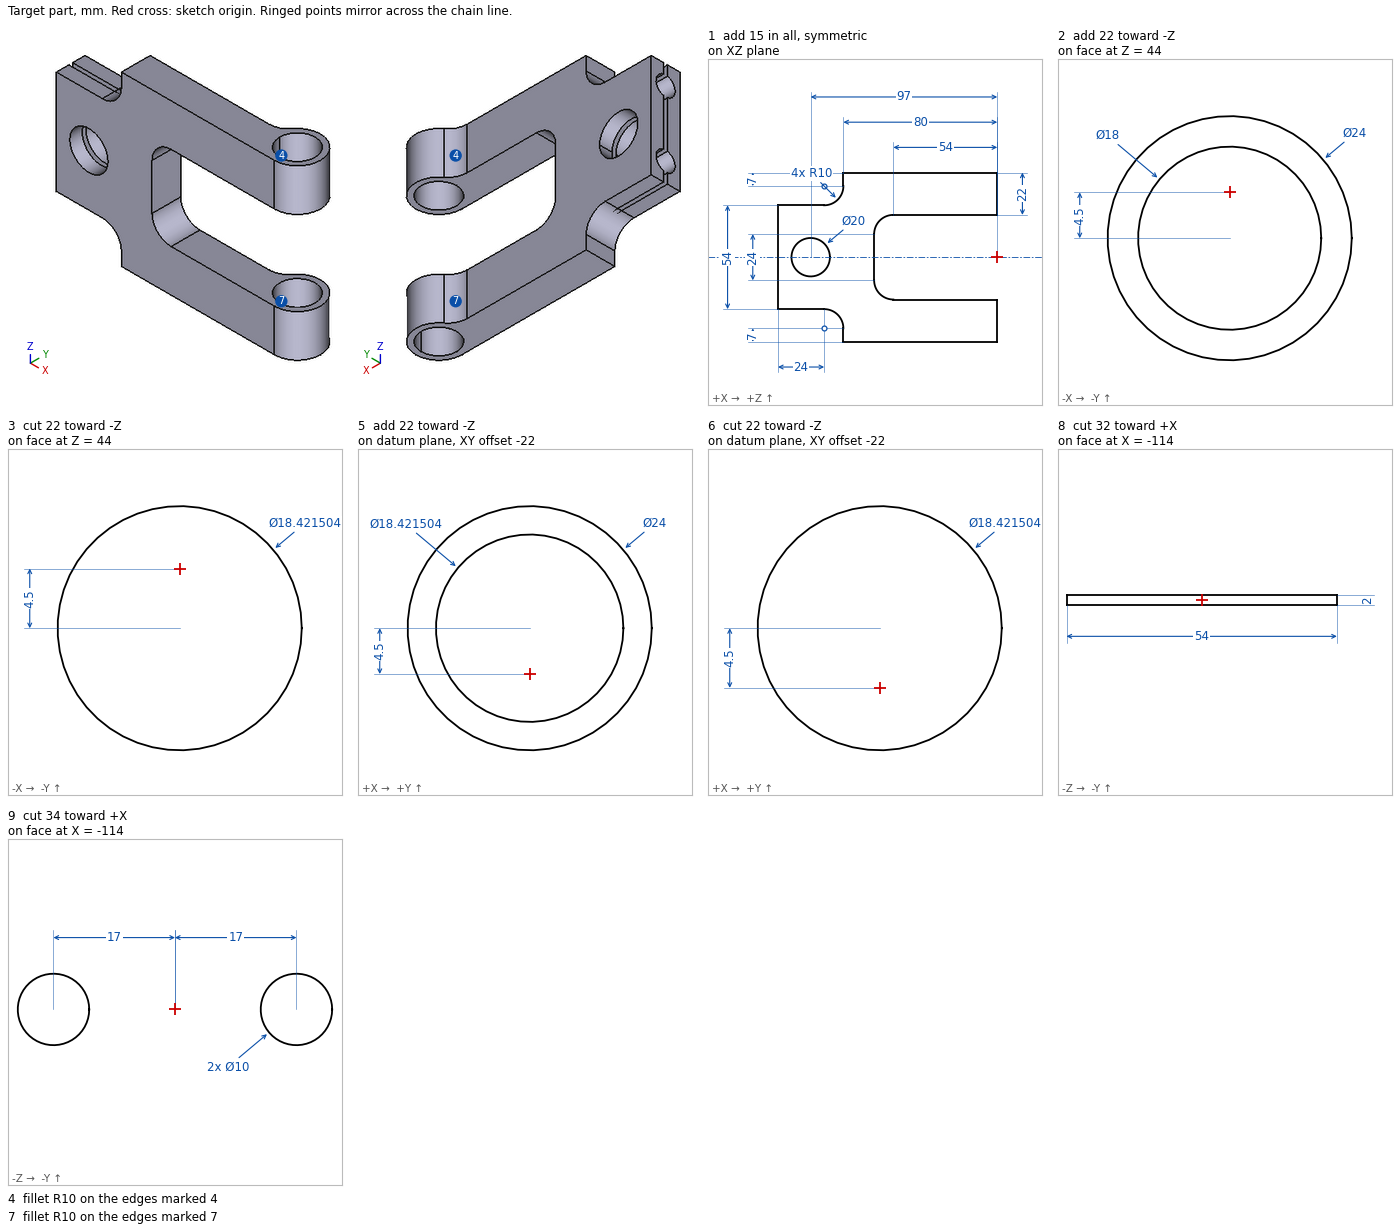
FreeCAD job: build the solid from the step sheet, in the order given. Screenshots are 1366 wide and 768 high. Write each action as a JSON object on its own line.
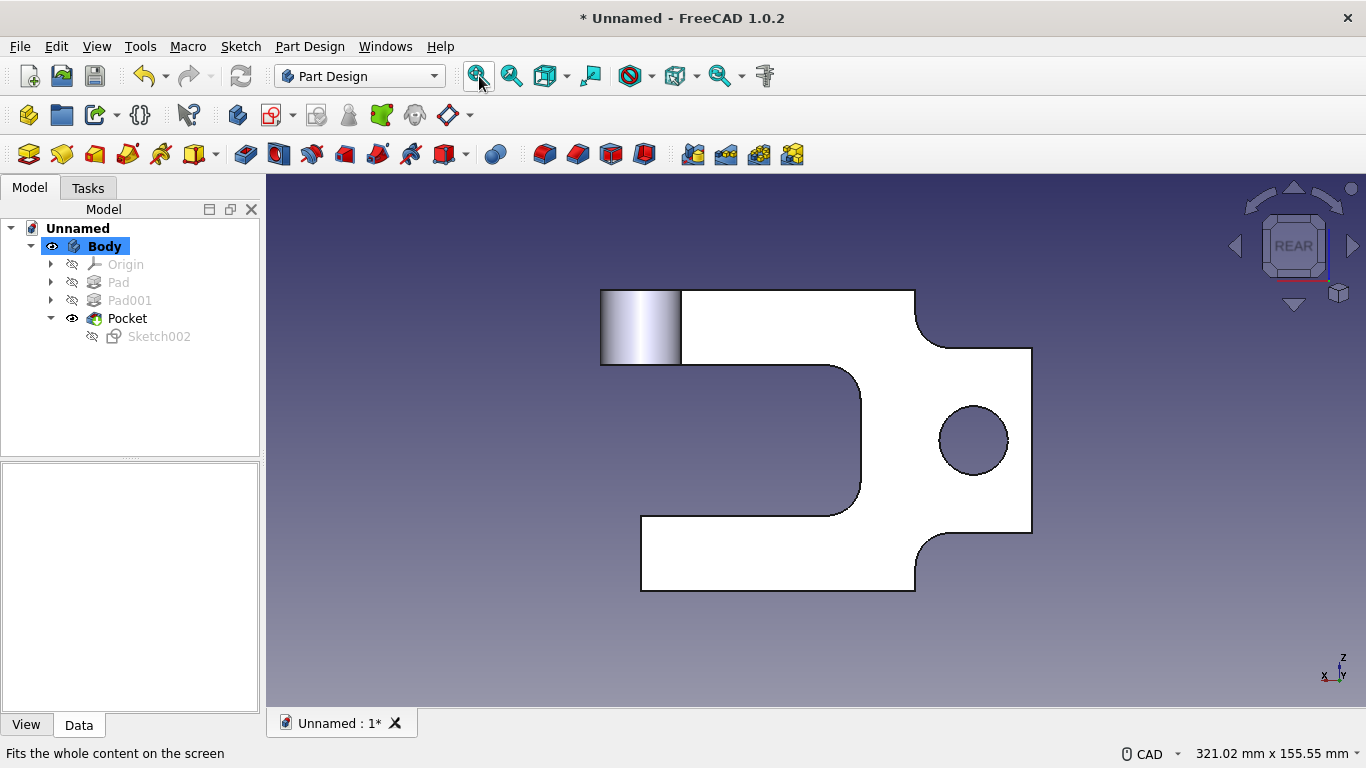
{"action": "key", "text": "6"}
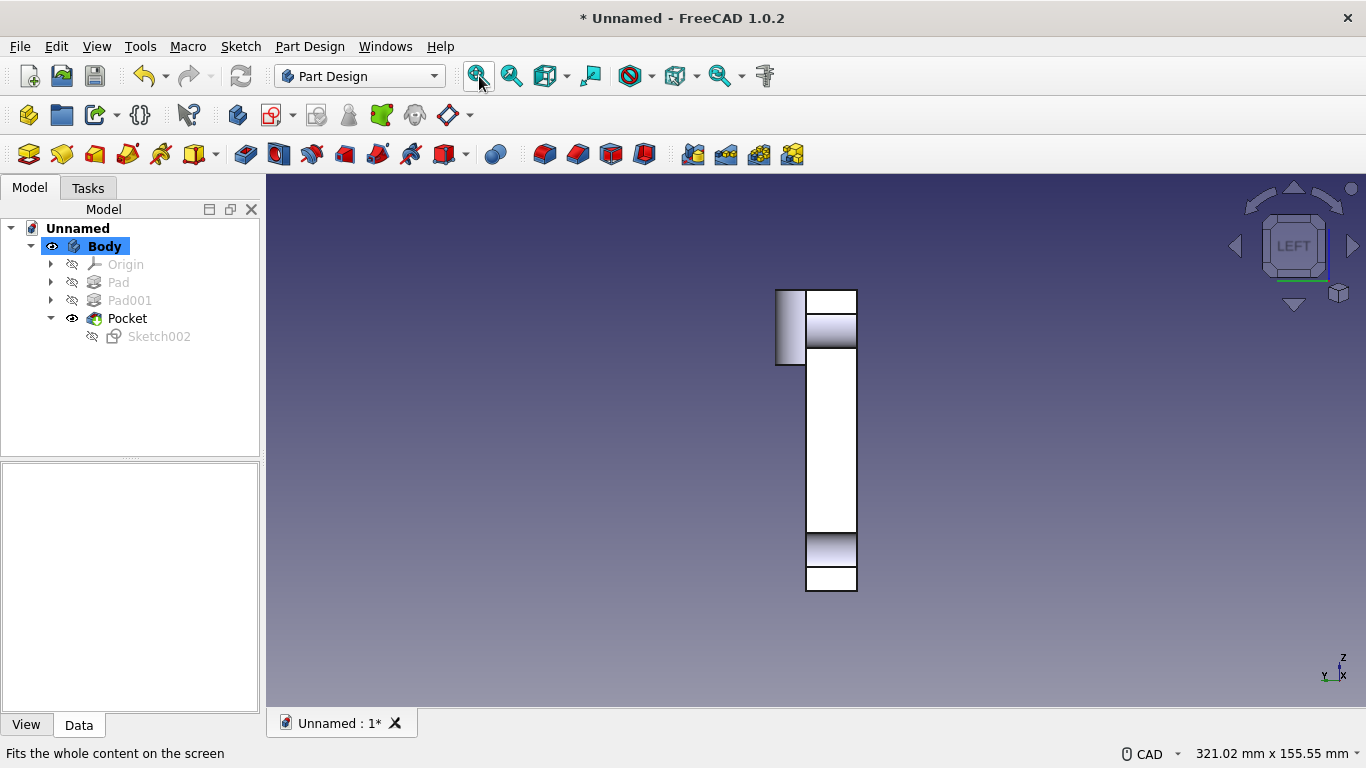
{"action": "key", "text": "v 3"}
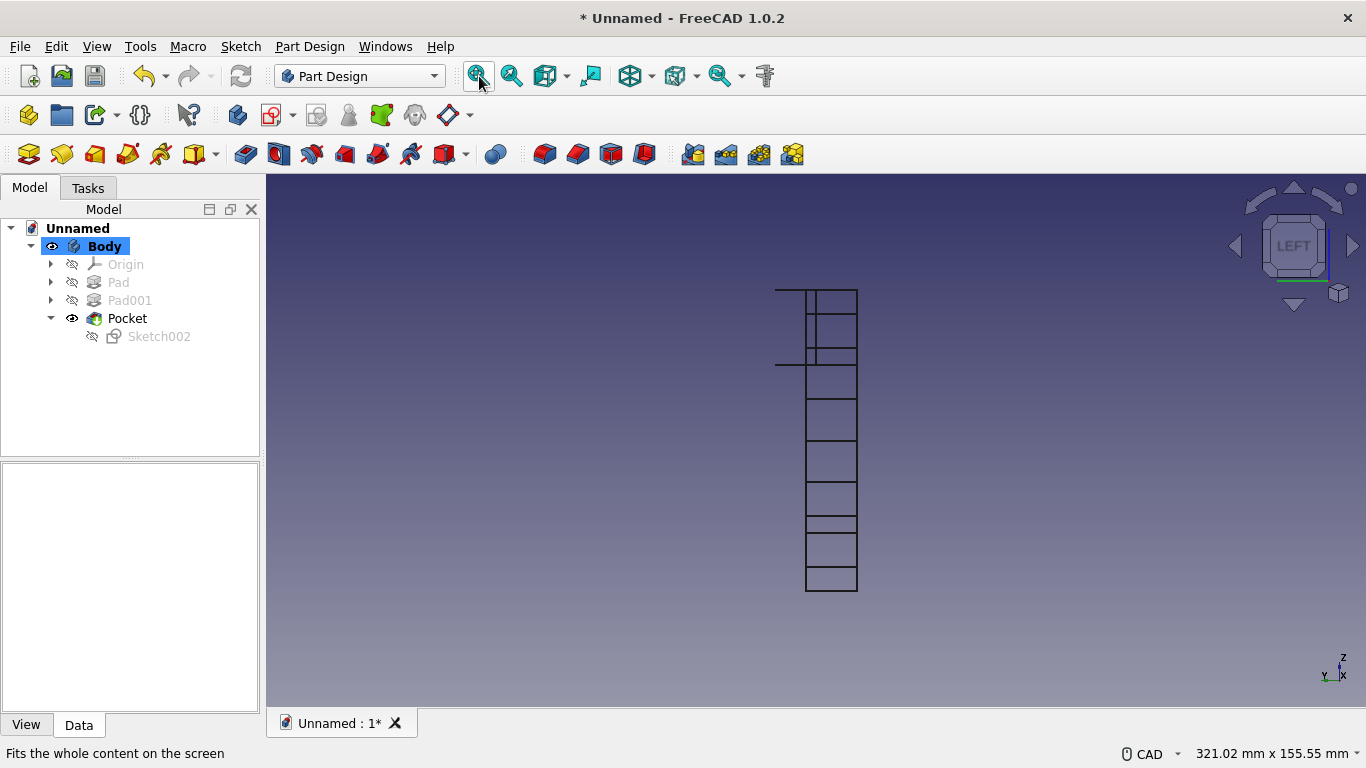
{"action": "key", "text": "0"}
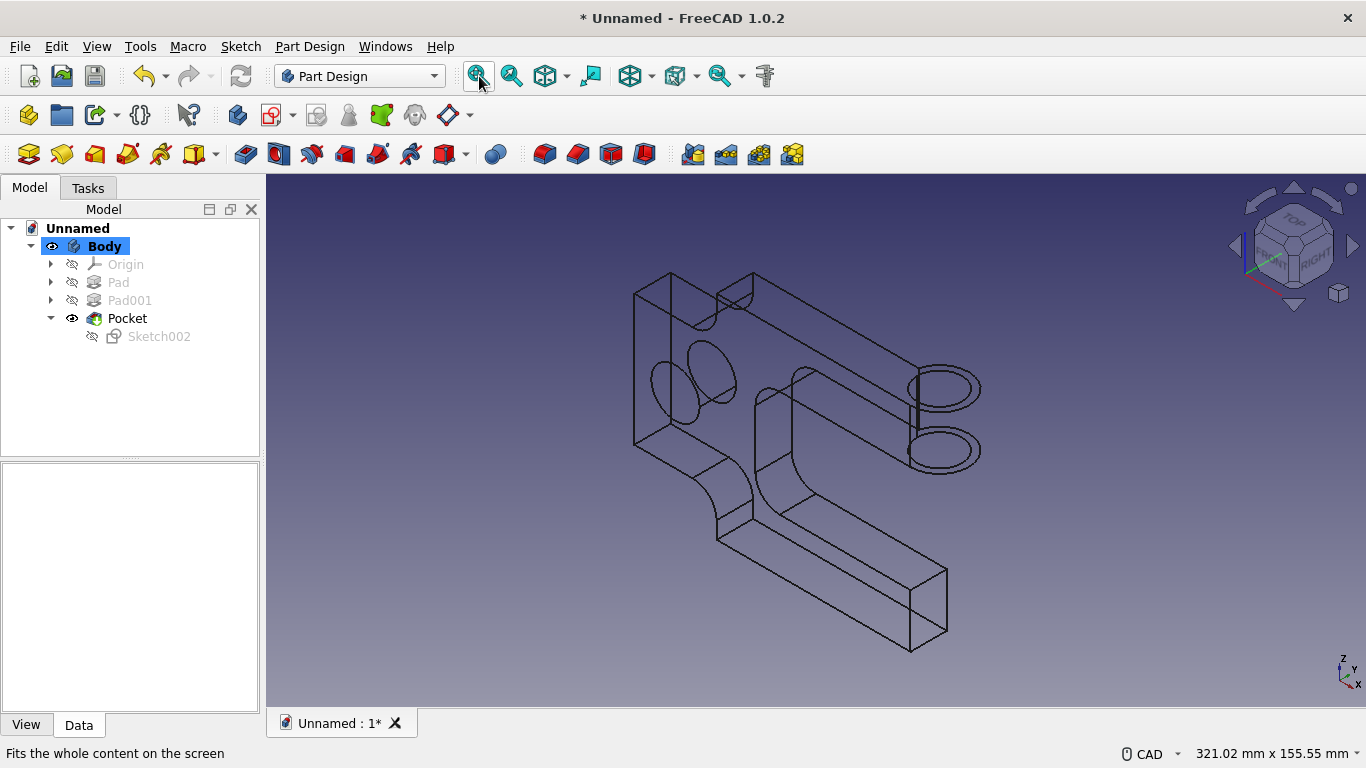
{"action": "key", "text": "2"}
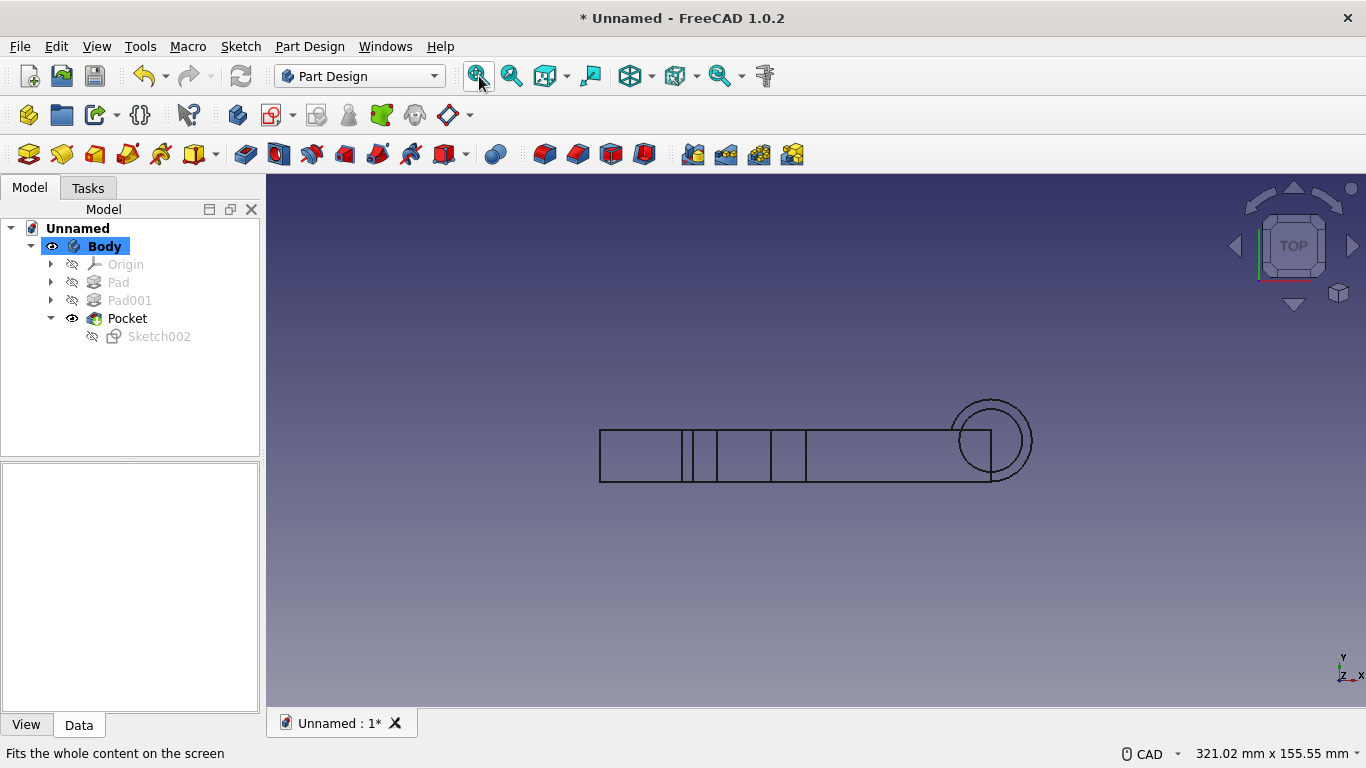
{"action": "left_click", "coordinate": [479, 76]}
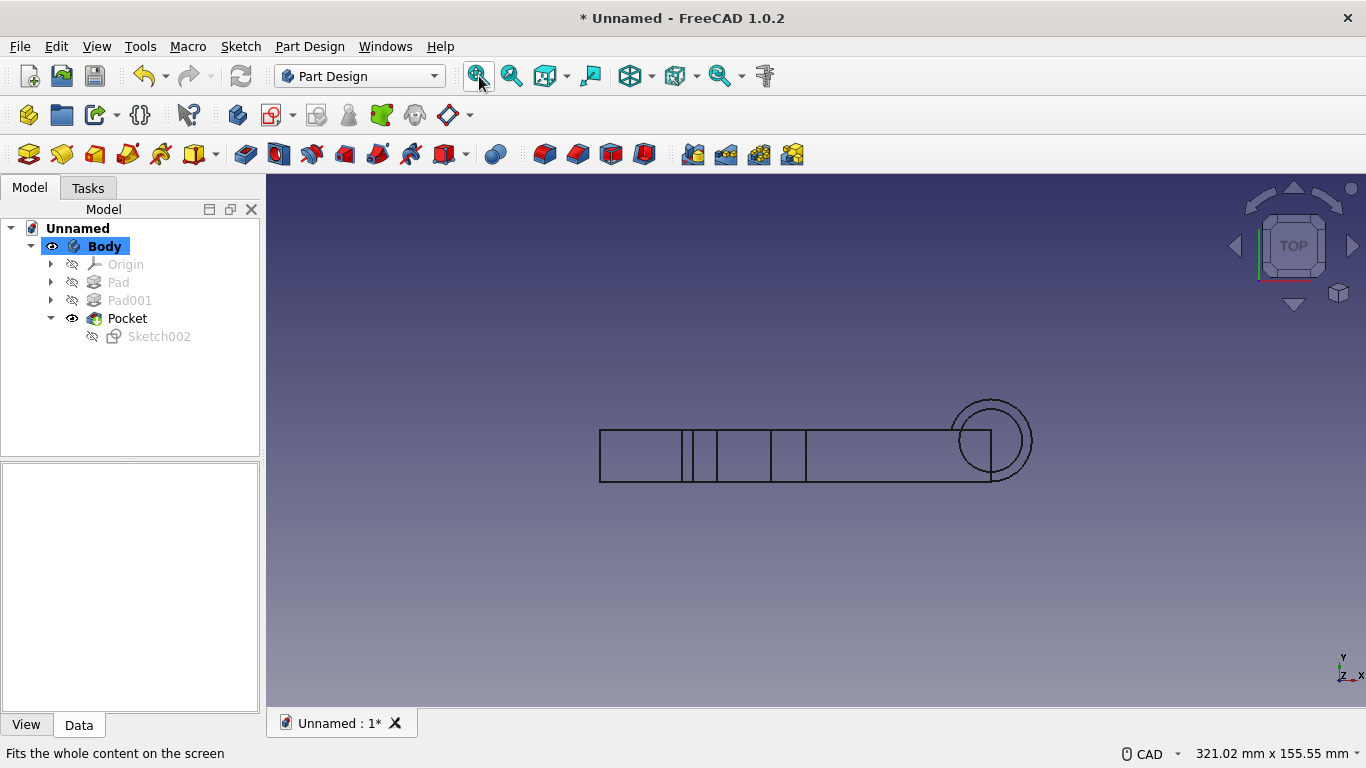
{"action": "key", "text": "1"}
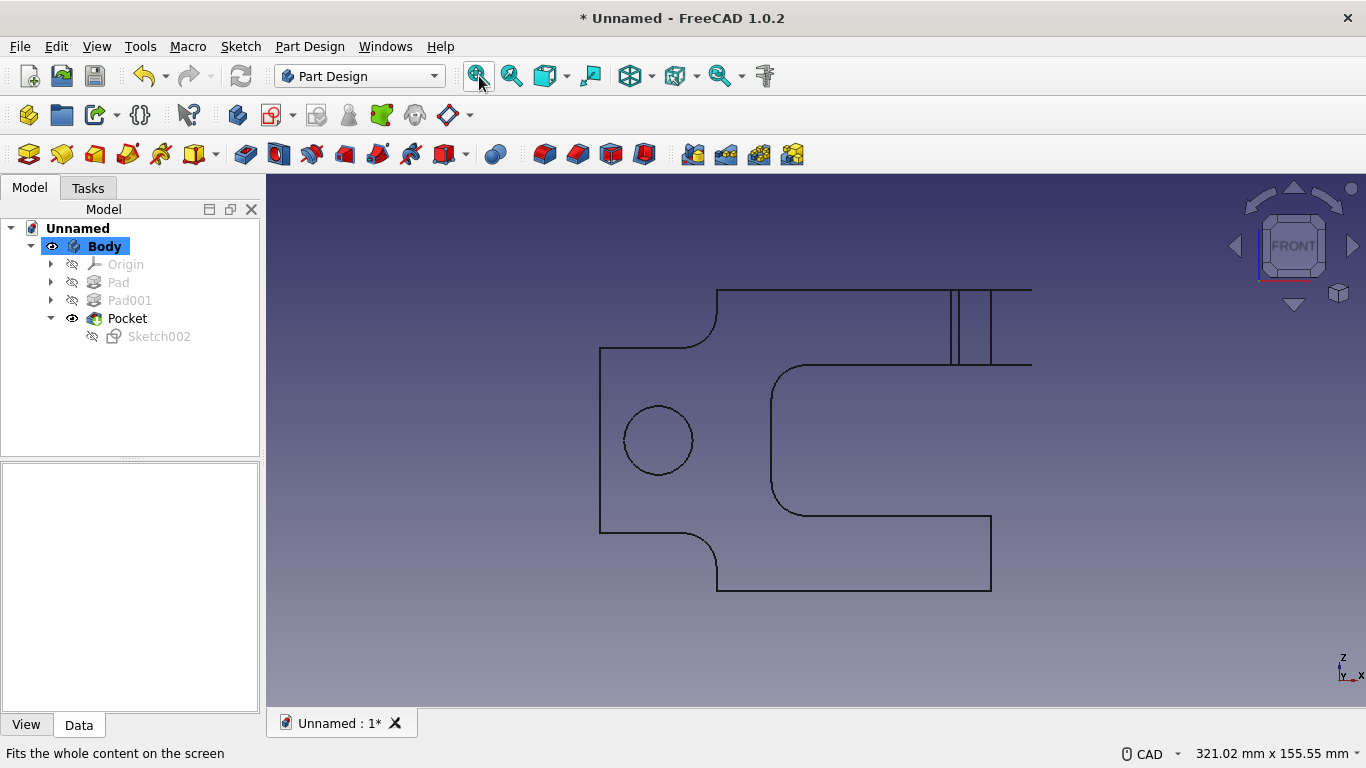
{"action": "left_click", "coordinate": [951, 326]}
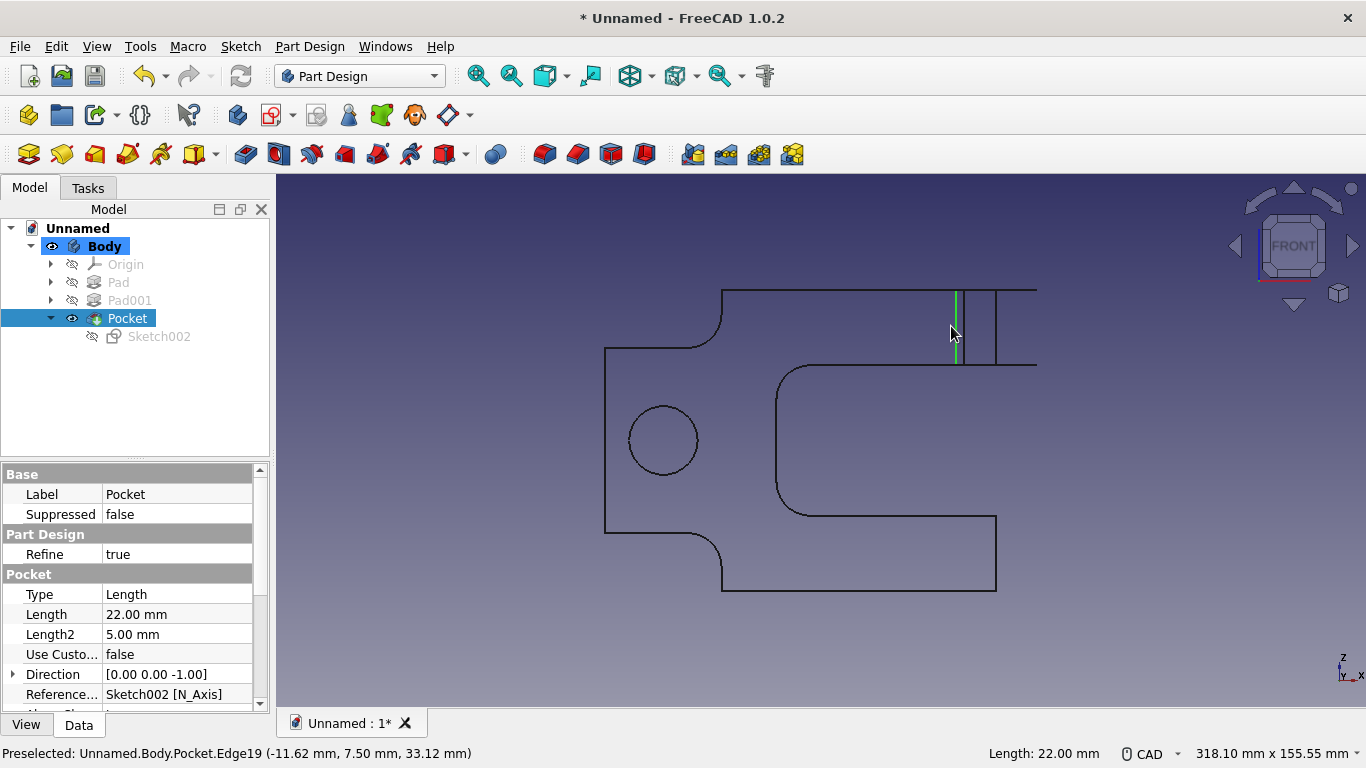
{"action": "key", "text": "v 1"}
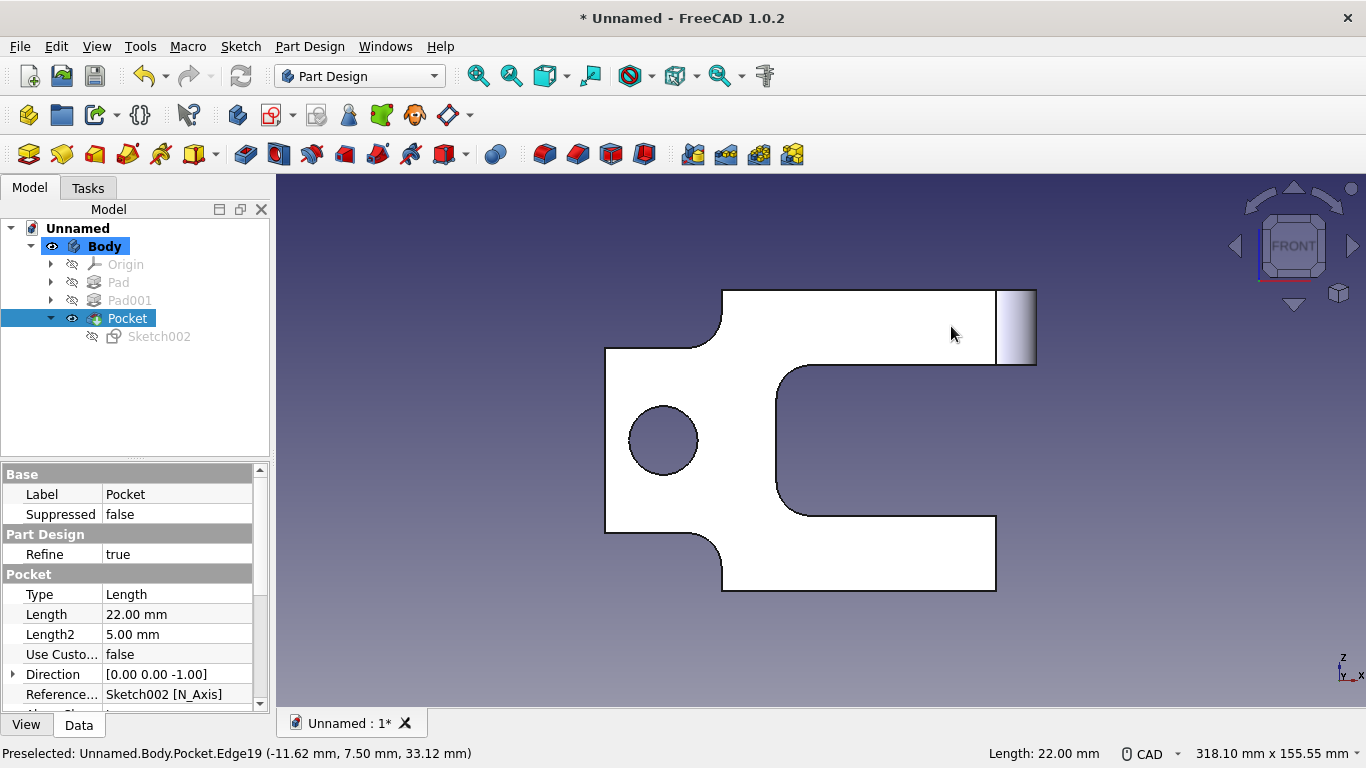
{"action": "left_click", "coordinate": [545, 154]}